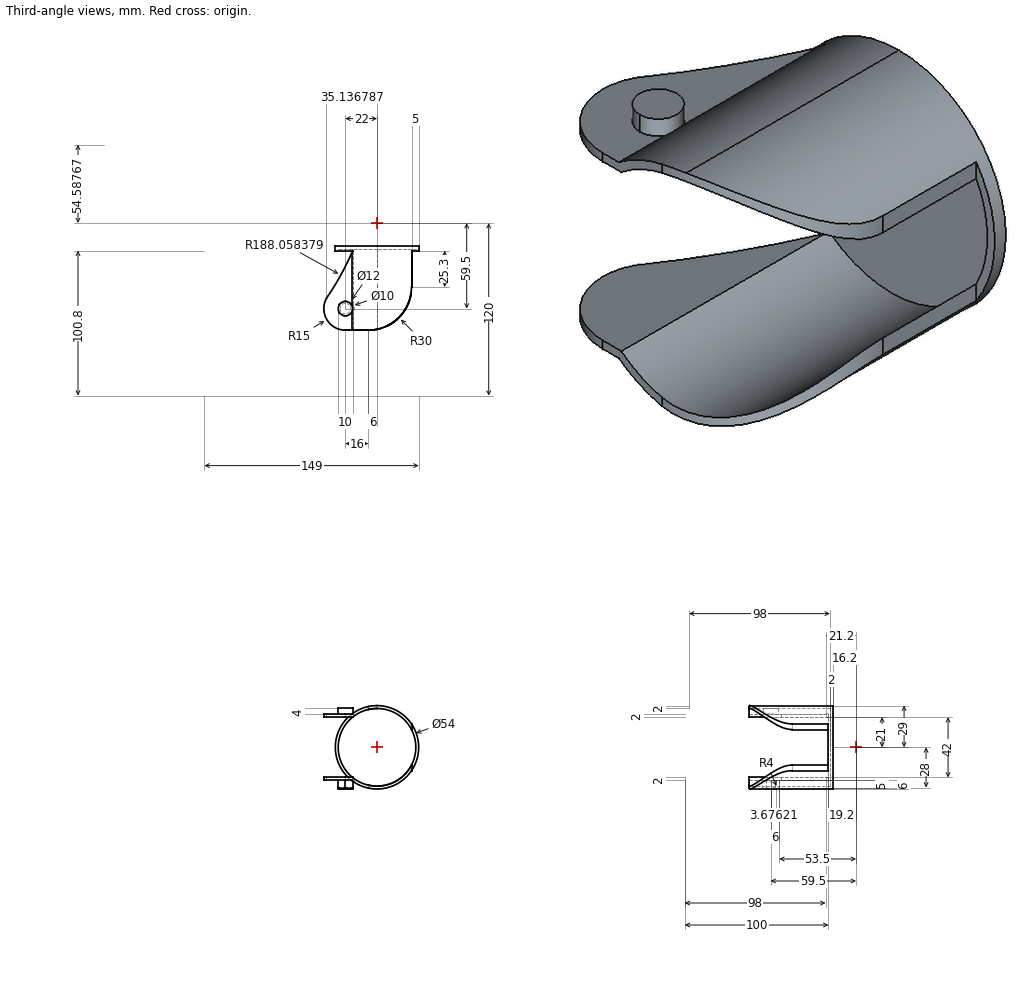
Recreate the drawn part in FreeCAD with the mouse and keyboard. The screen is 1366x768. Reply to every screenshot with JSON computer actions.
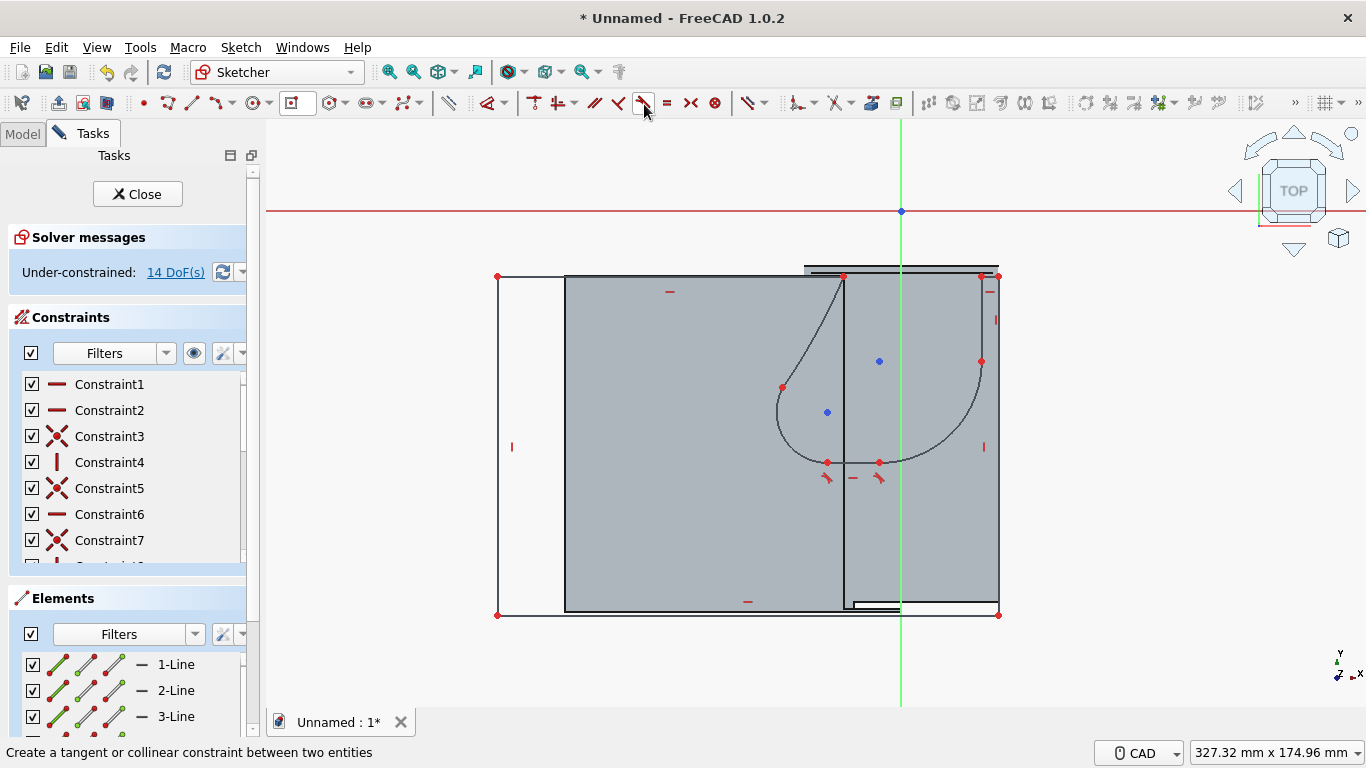
{"action": "left_click", "coordinate": [982, 302]}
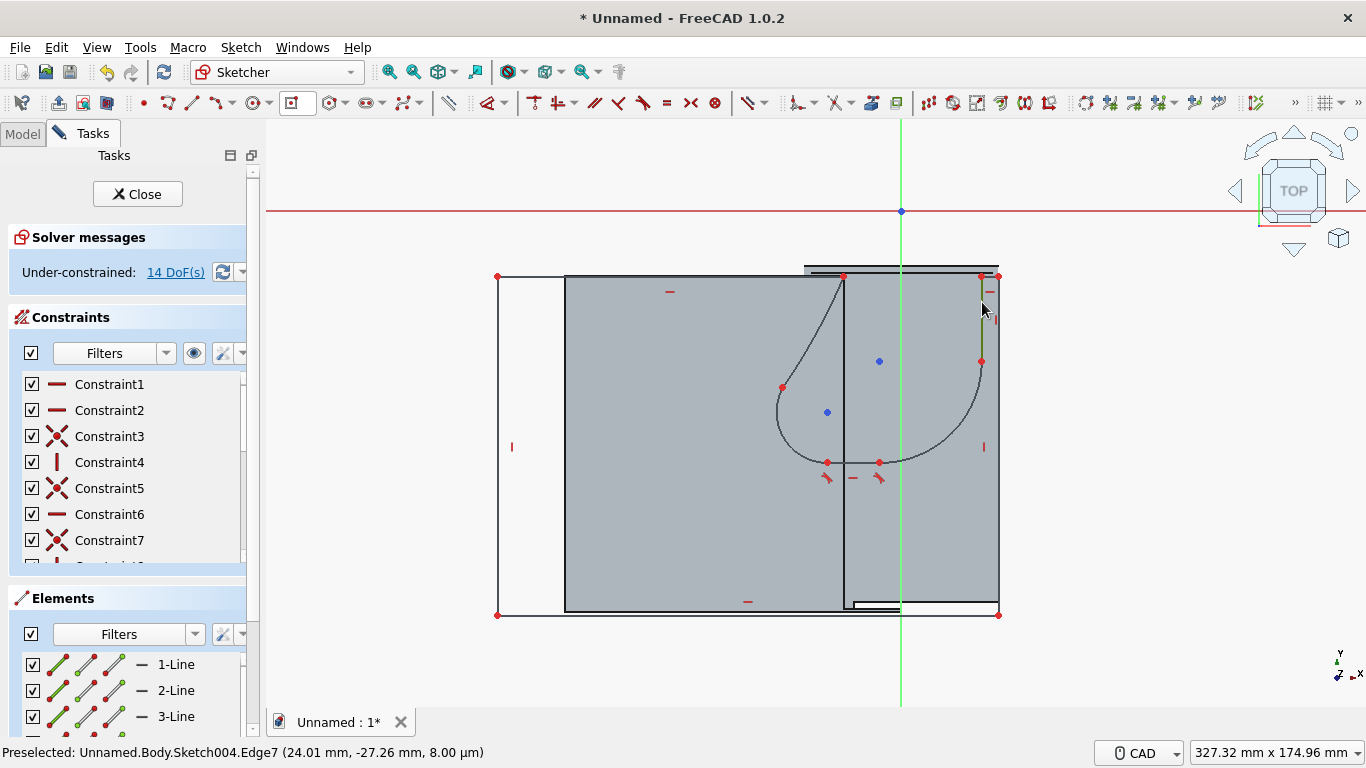
{"action": "left_click", "coordinate": [926, 452]}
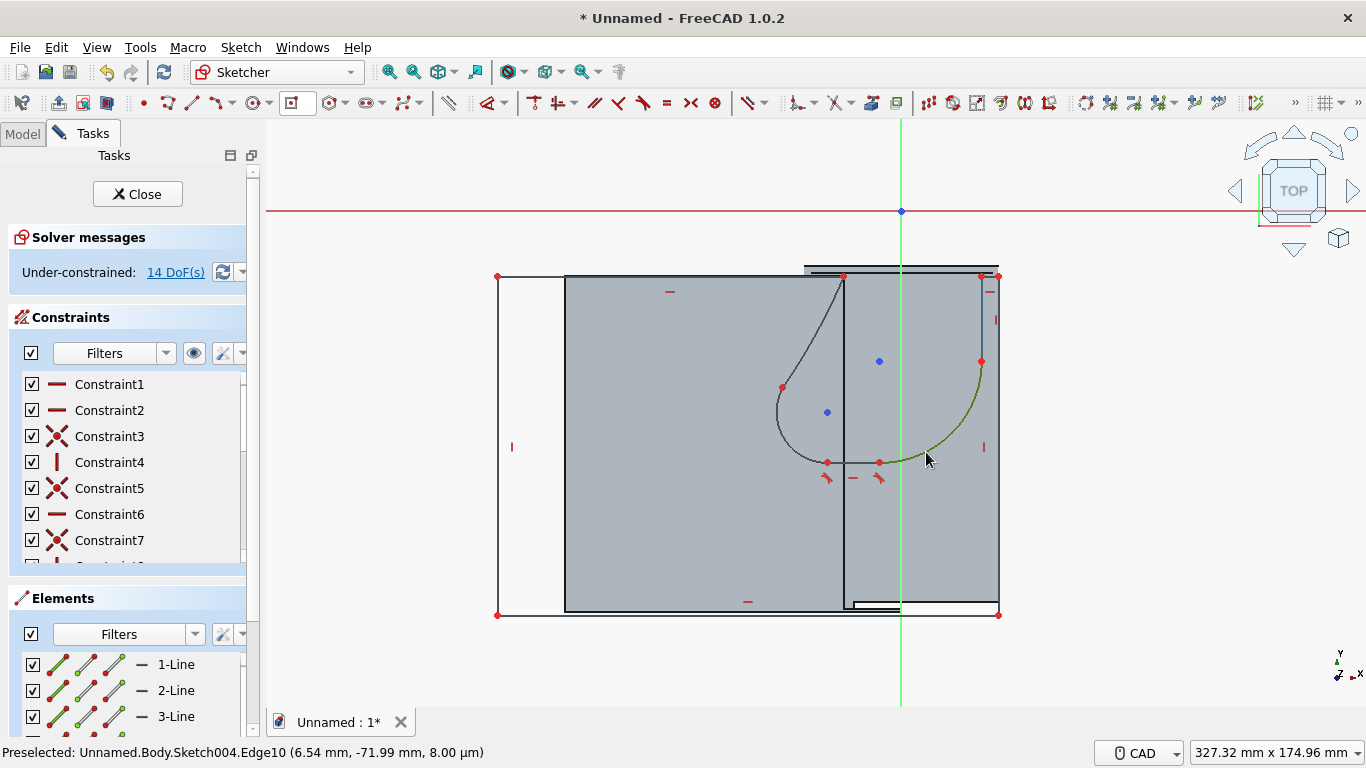
{"action": "left_click", "coordinate": [644, 104]}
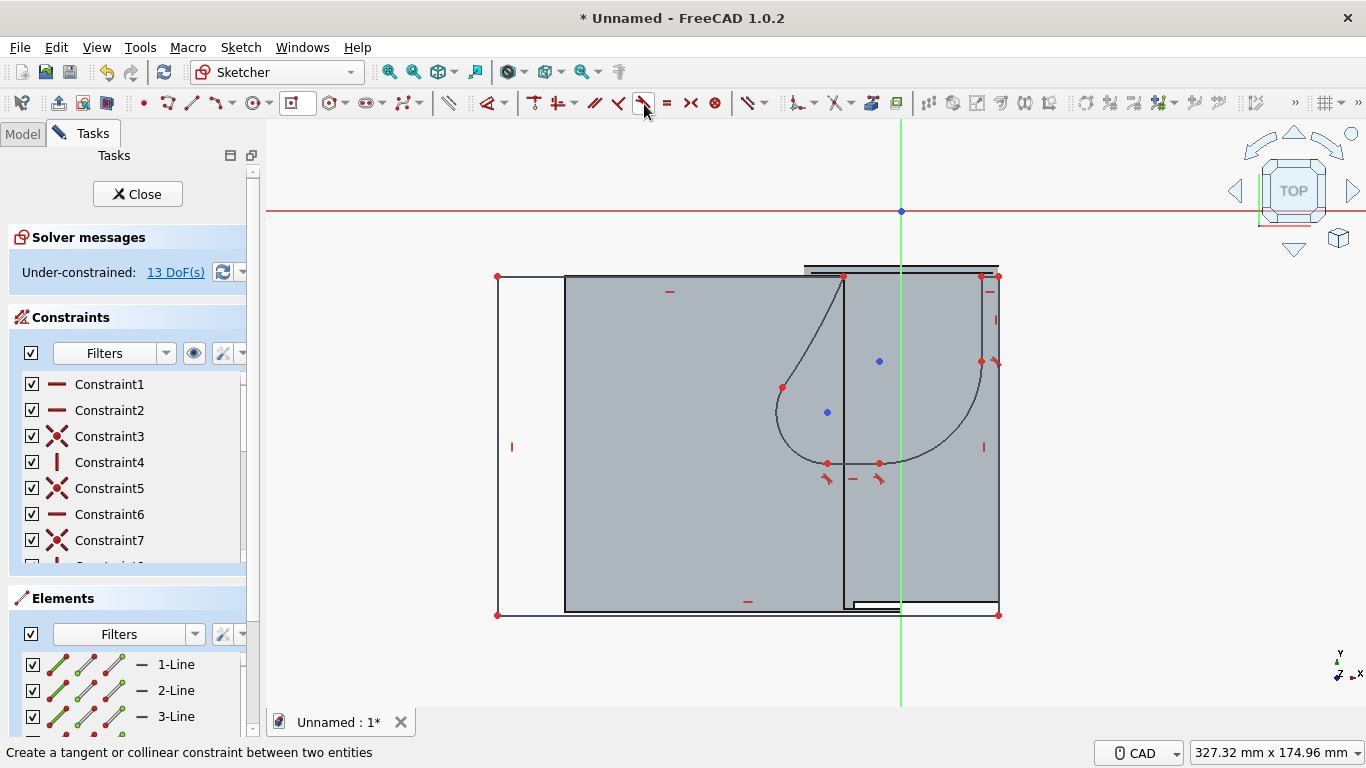
{"action": "left_click", "coordinate": [488, 104]}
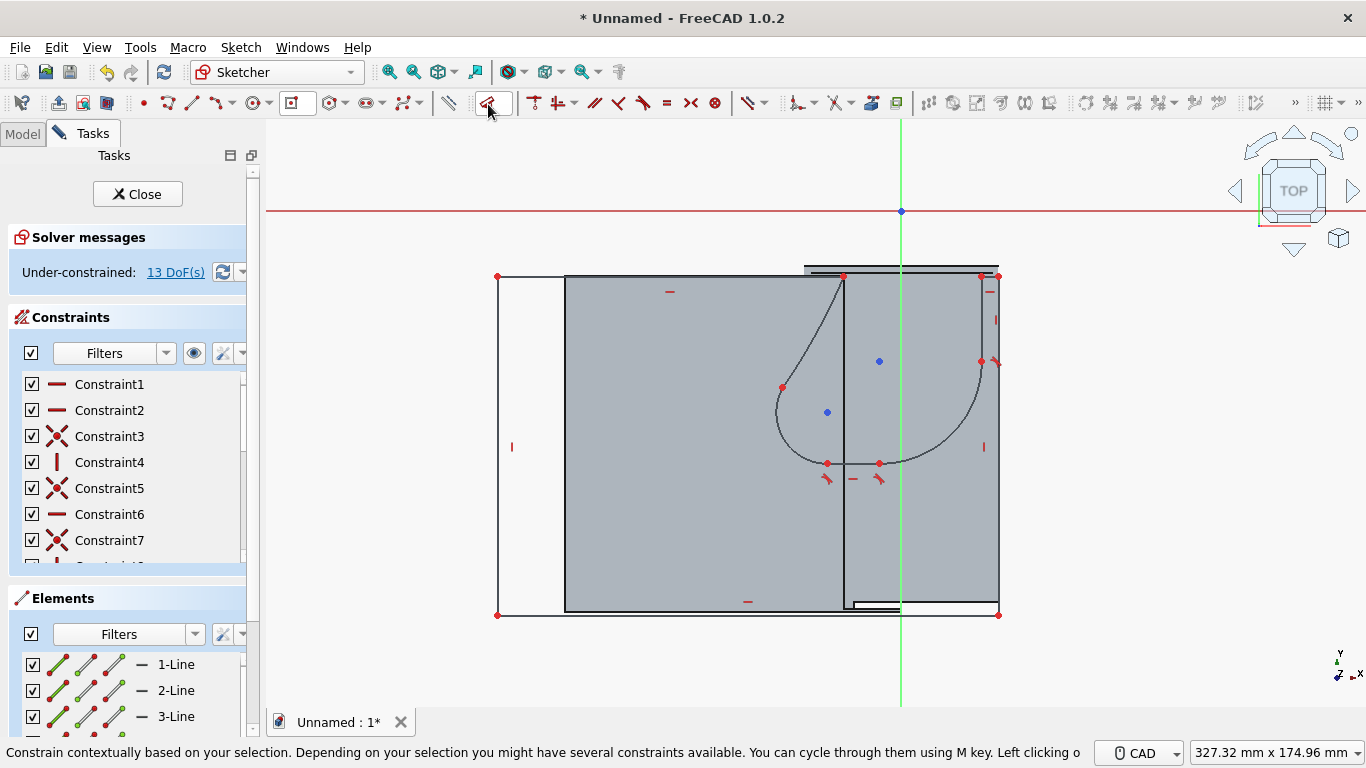
{"action": "left_click", "coordinate": [777, 419]}
{"action": "left_click", "coordinate": [745, 423]}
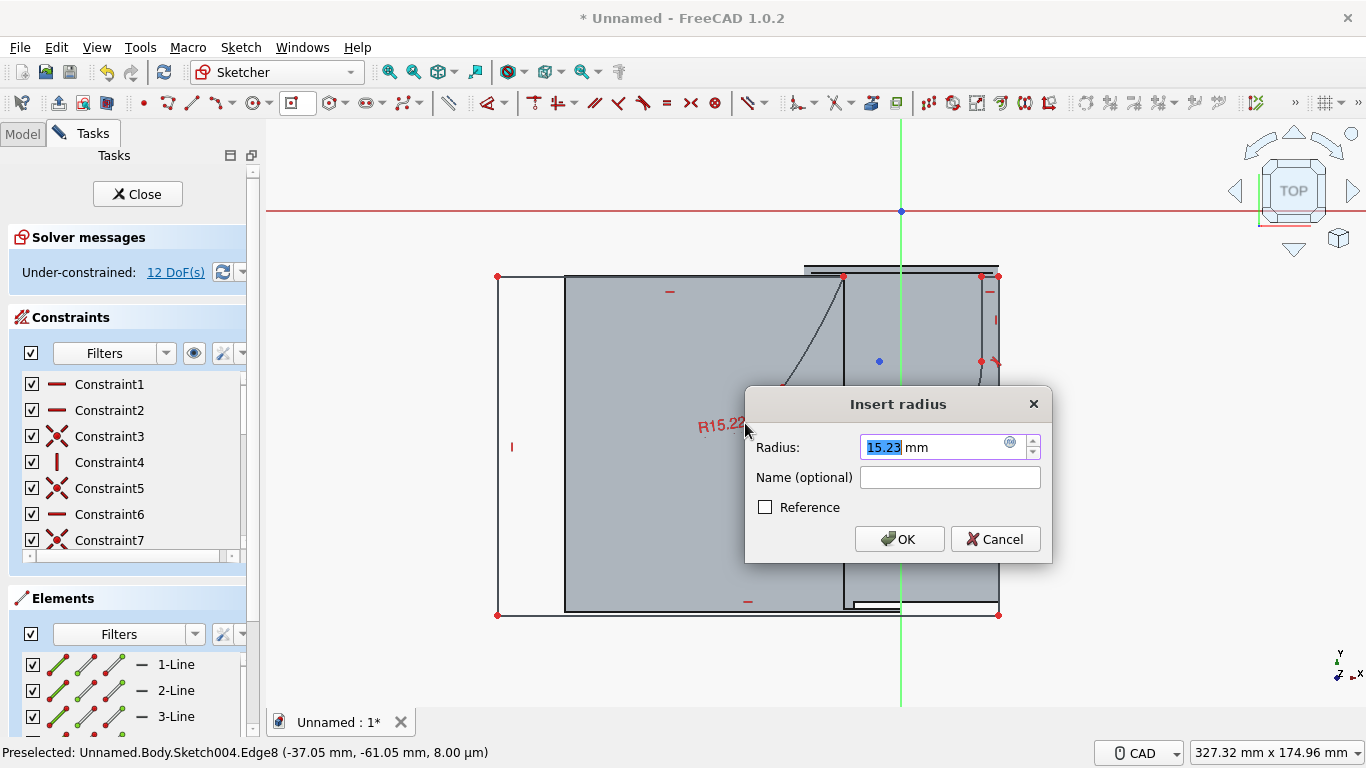
{"action": "type", "text": "15"}
{"action": "key", "text": "Return"}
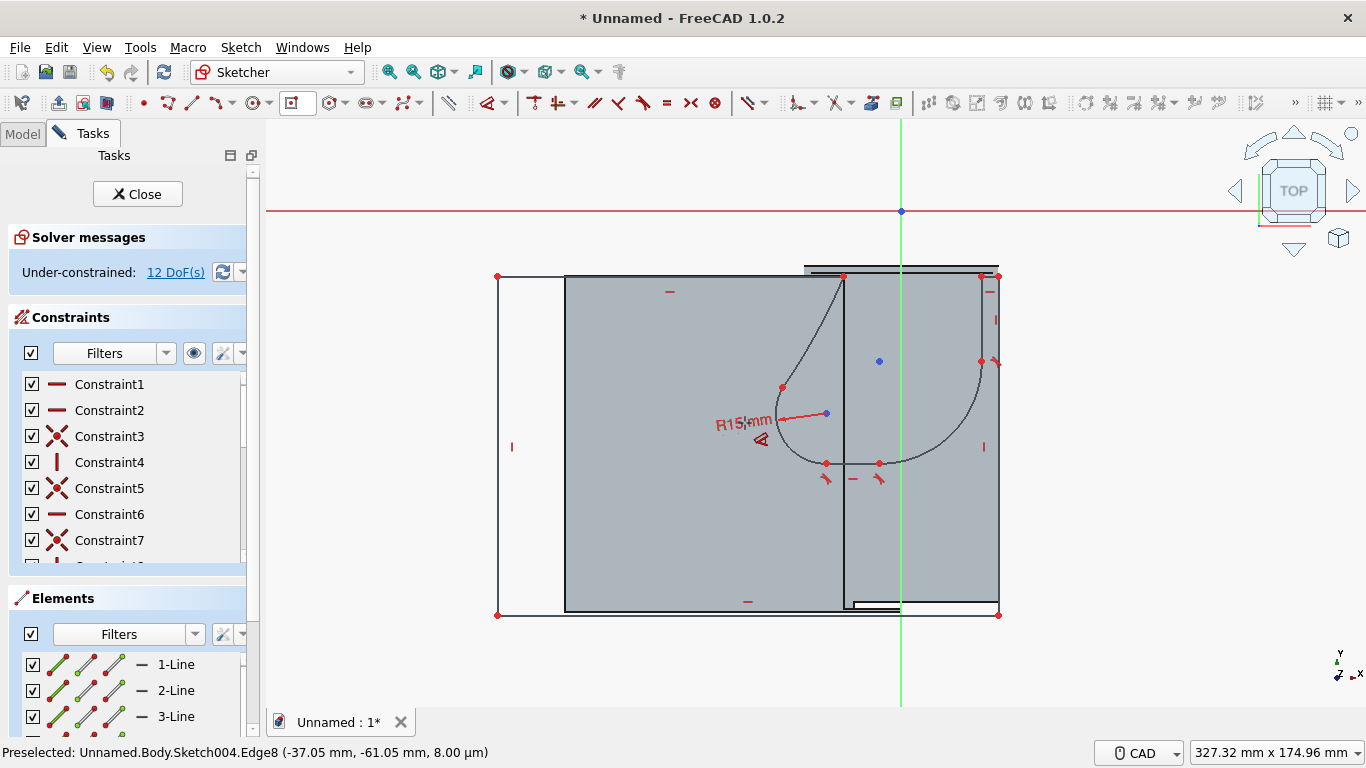
{"action": "left_click", "coordinate": [803, 356]}
{"action": "left_click", "coordinate": [830, 373]}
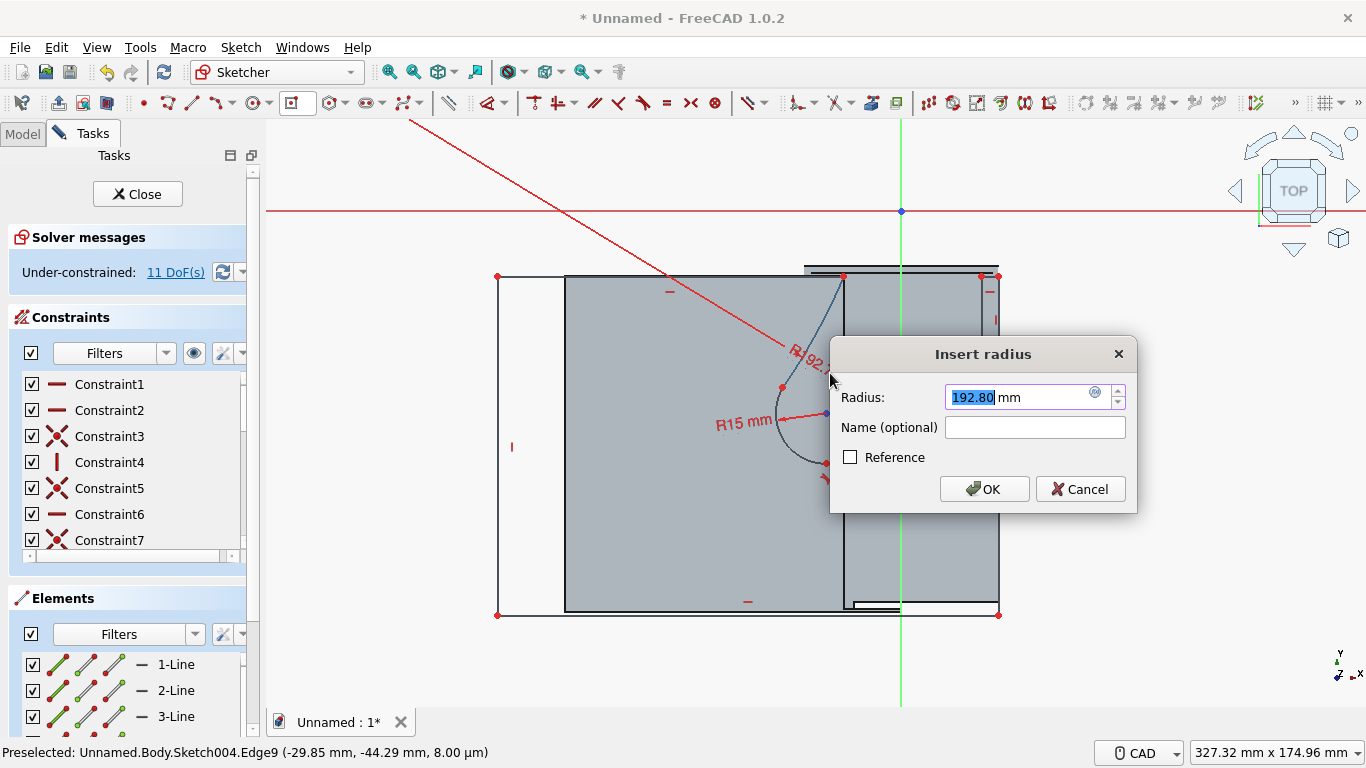
{"action": "type", "text": "188.058379"}
{"action": "key", "text": "Return"}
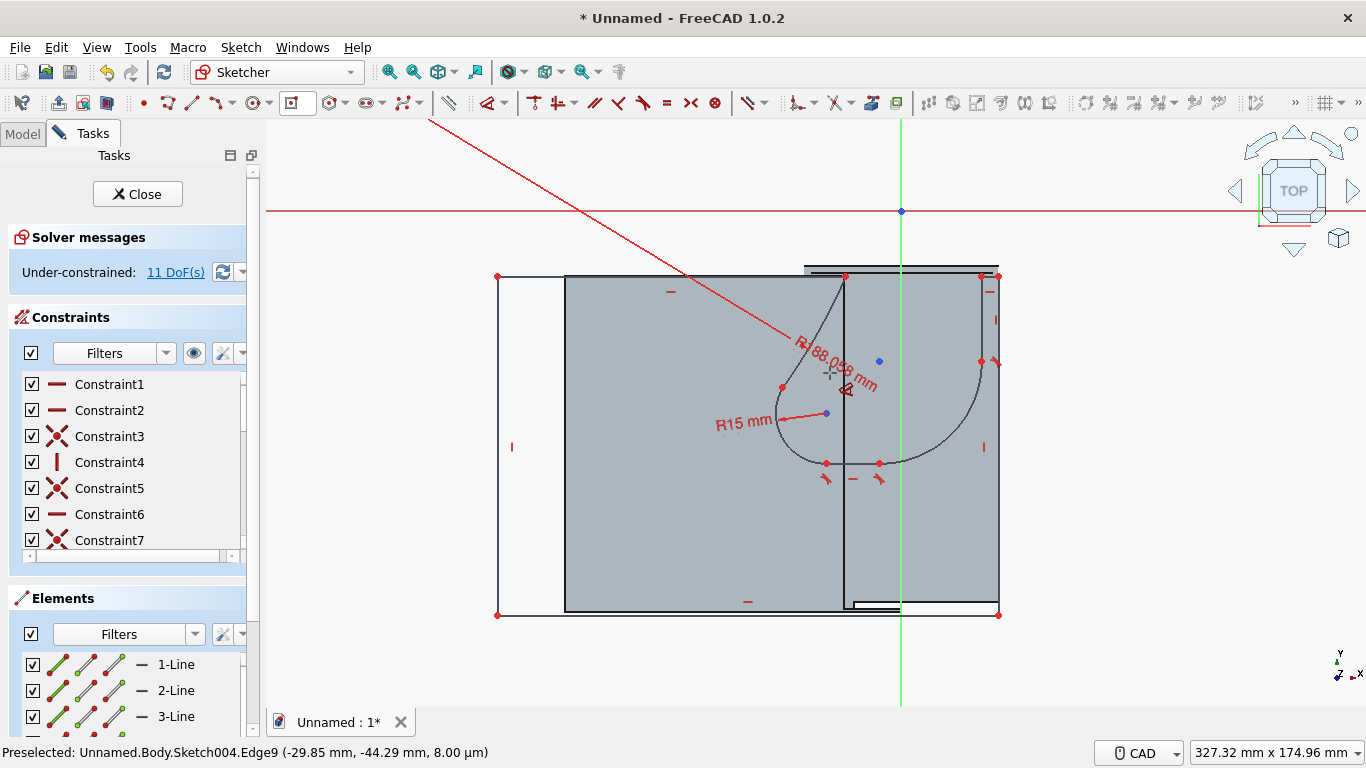
{"action": "left_click", "coordinate": [926, 453]}
{"action": "left_click", "coordinate": [940, 482]}